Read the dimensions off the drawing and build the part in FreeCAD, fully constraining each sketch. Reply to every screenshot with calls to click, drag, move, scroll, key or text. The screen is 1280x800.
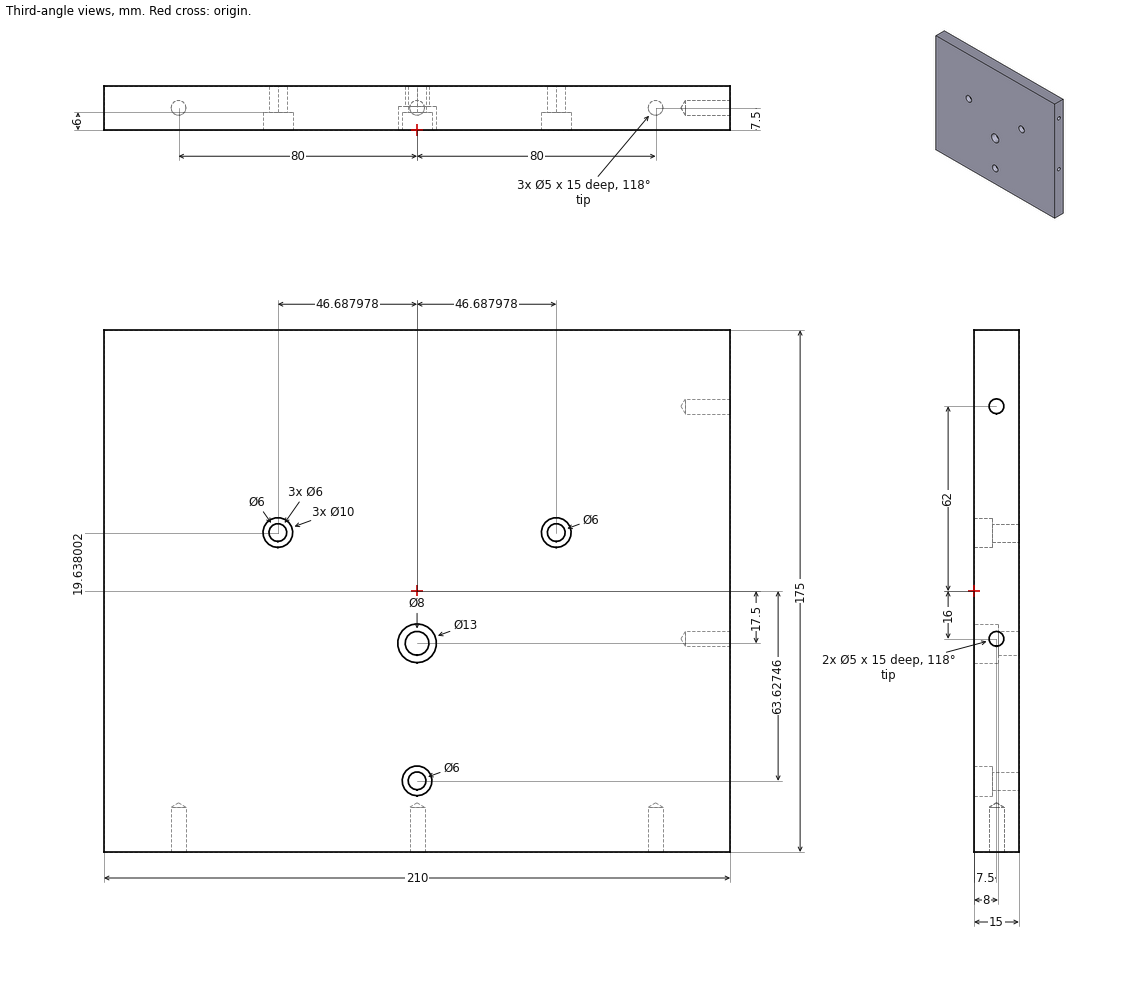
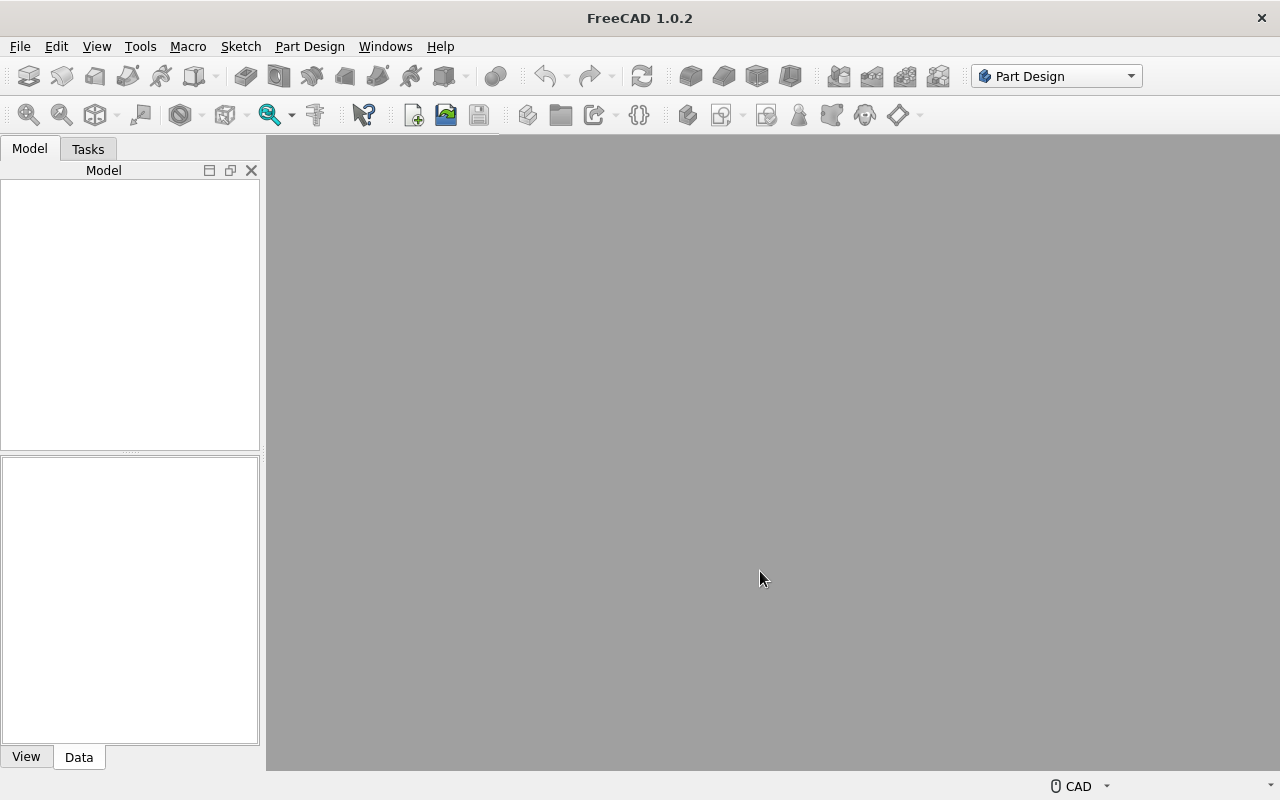
click(413, 116)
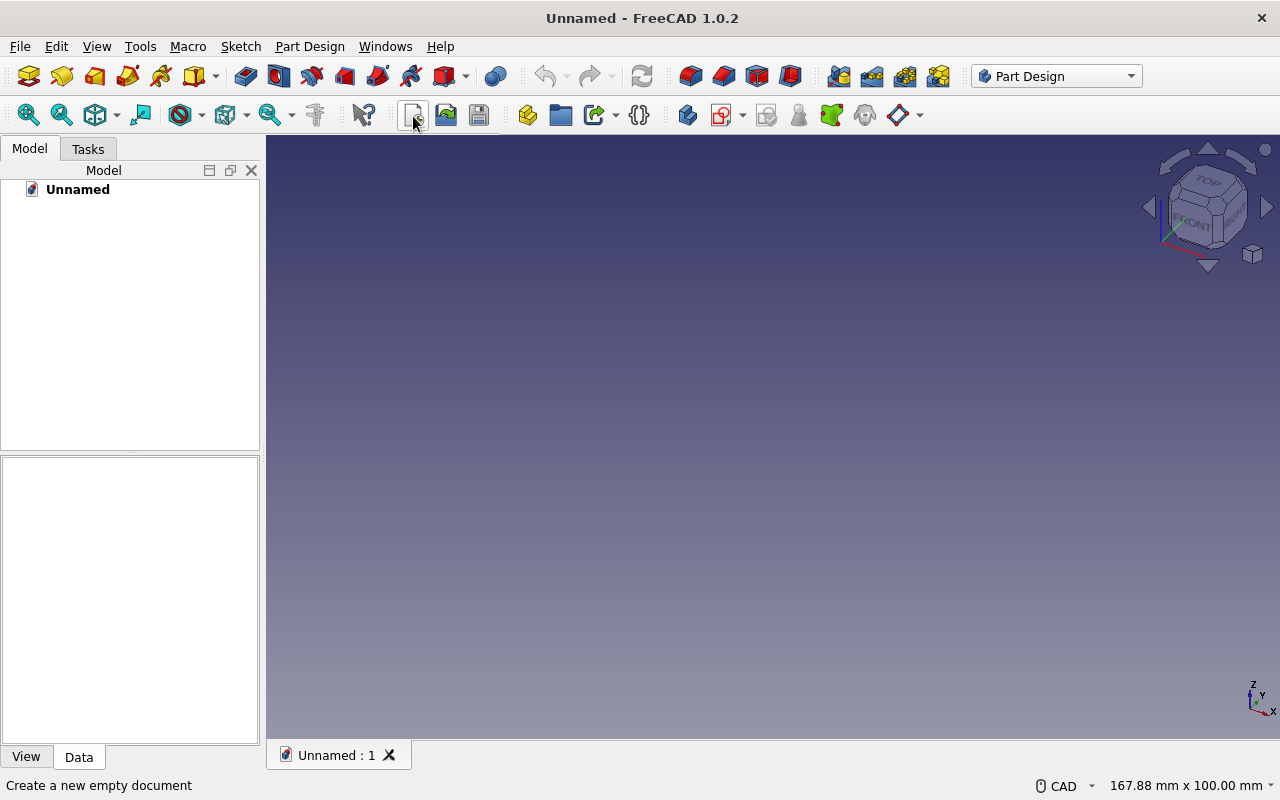
click(720, 116)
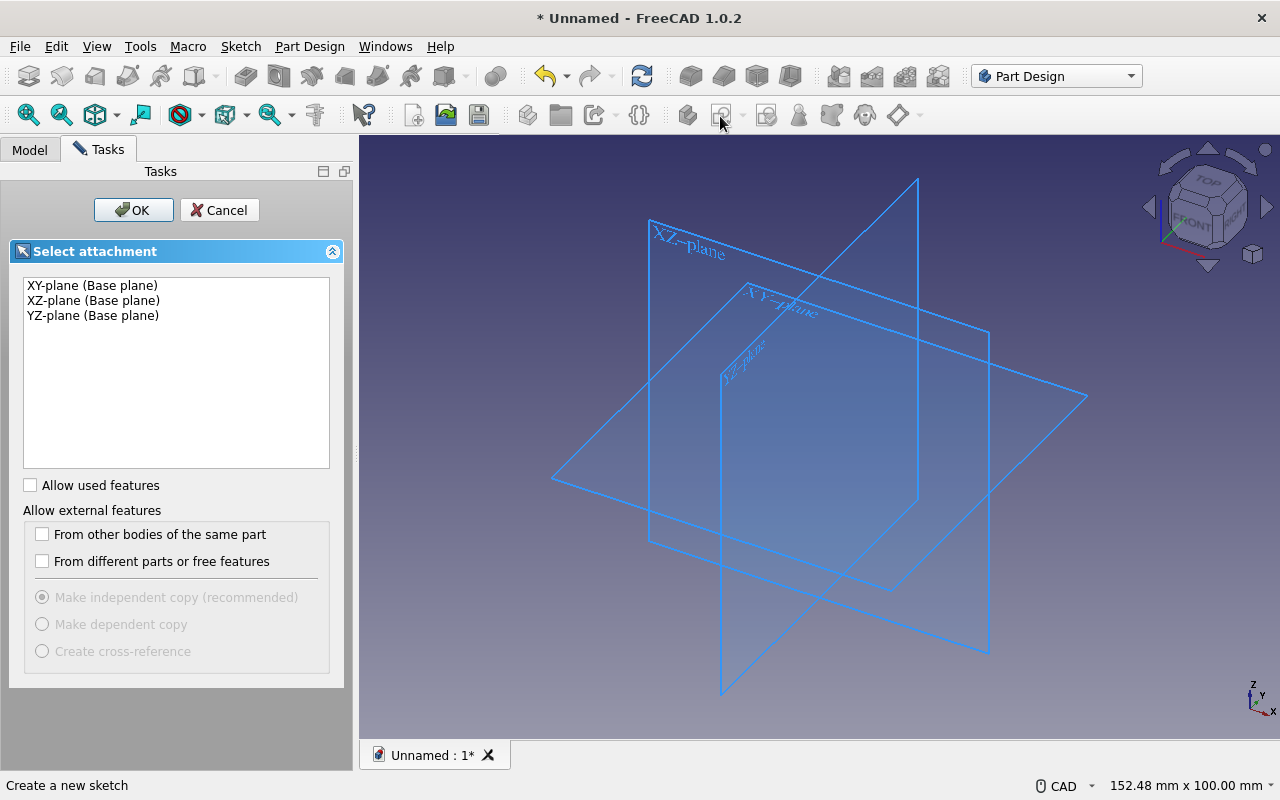
click(84, 300)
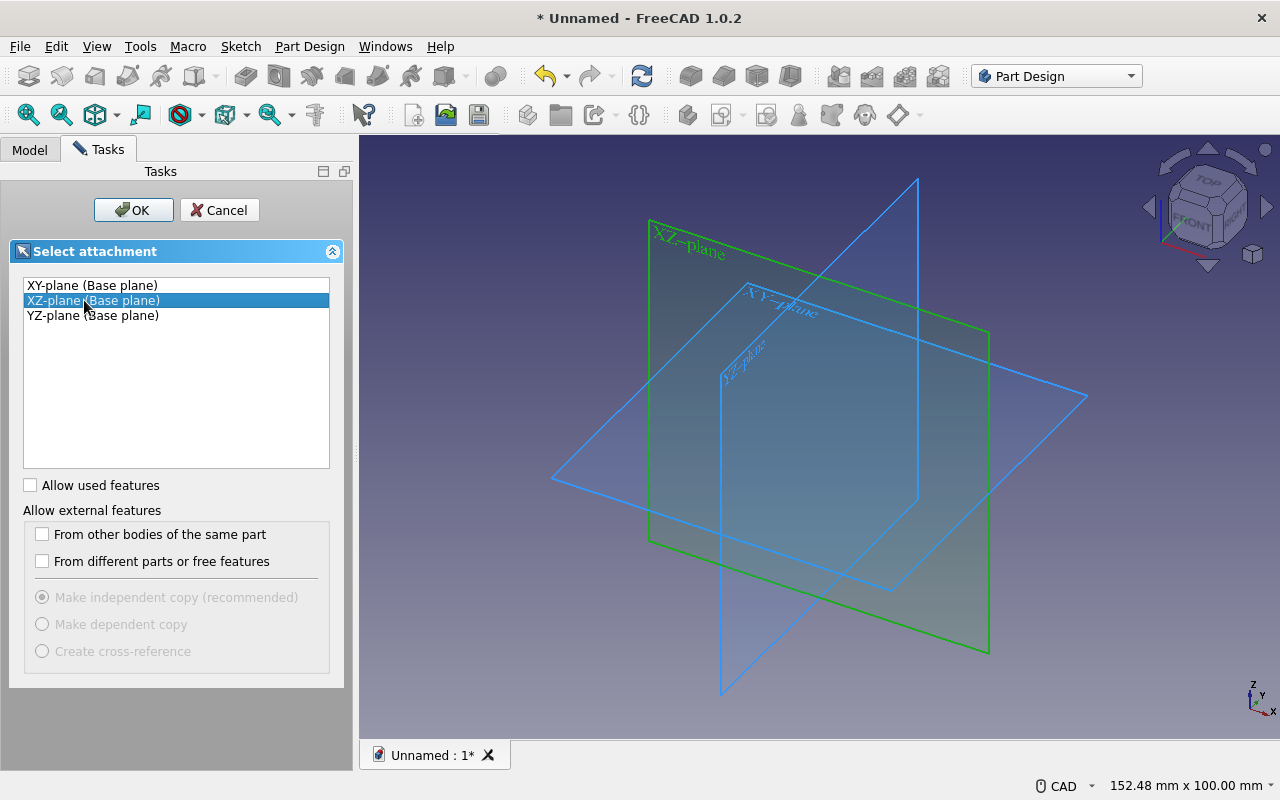
click(134, 210)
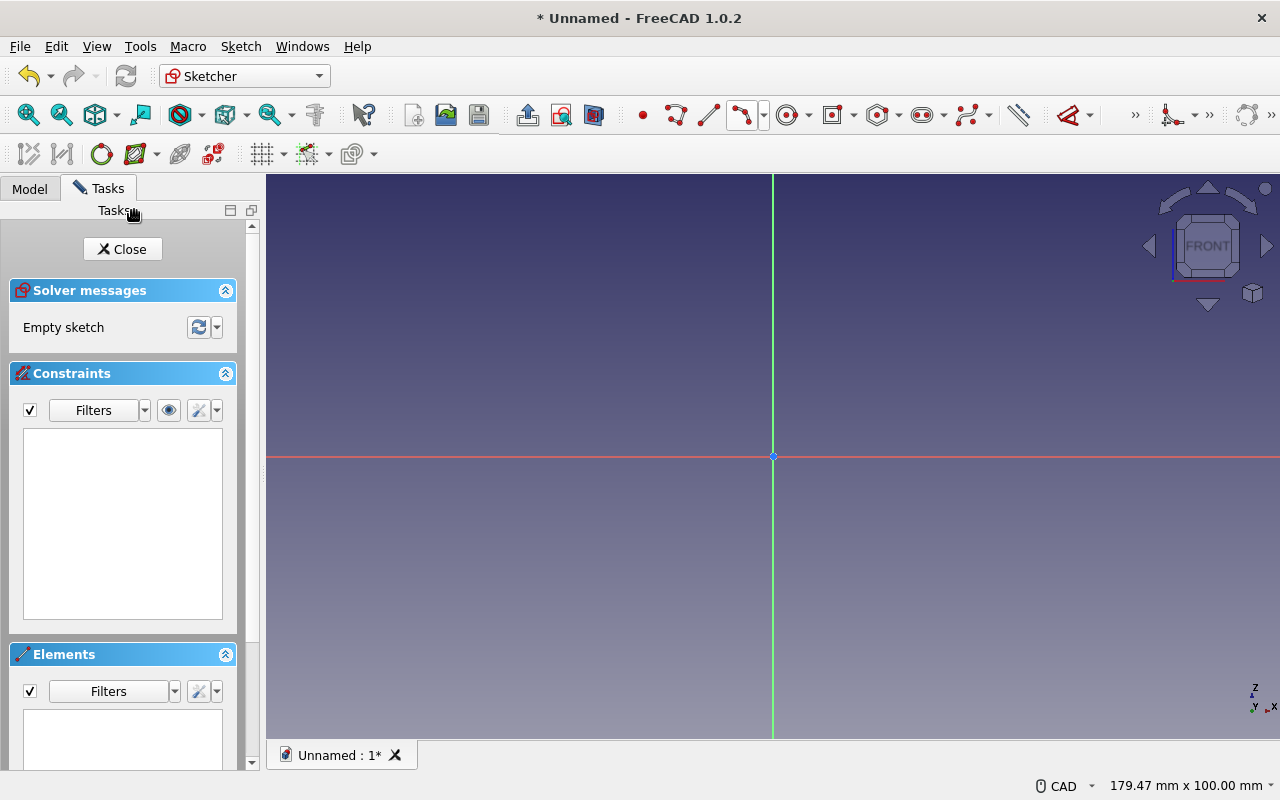
scroll(665, 456, down, 5)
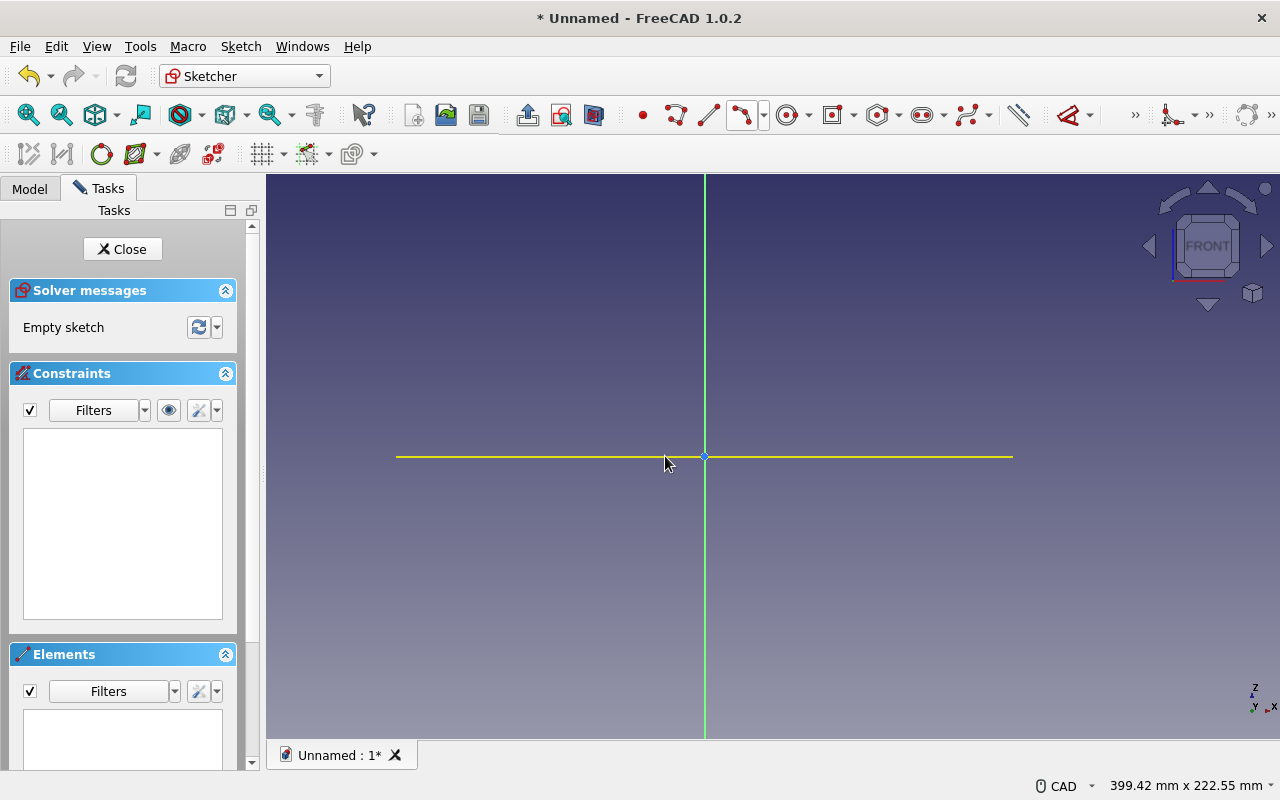
click(832, 116)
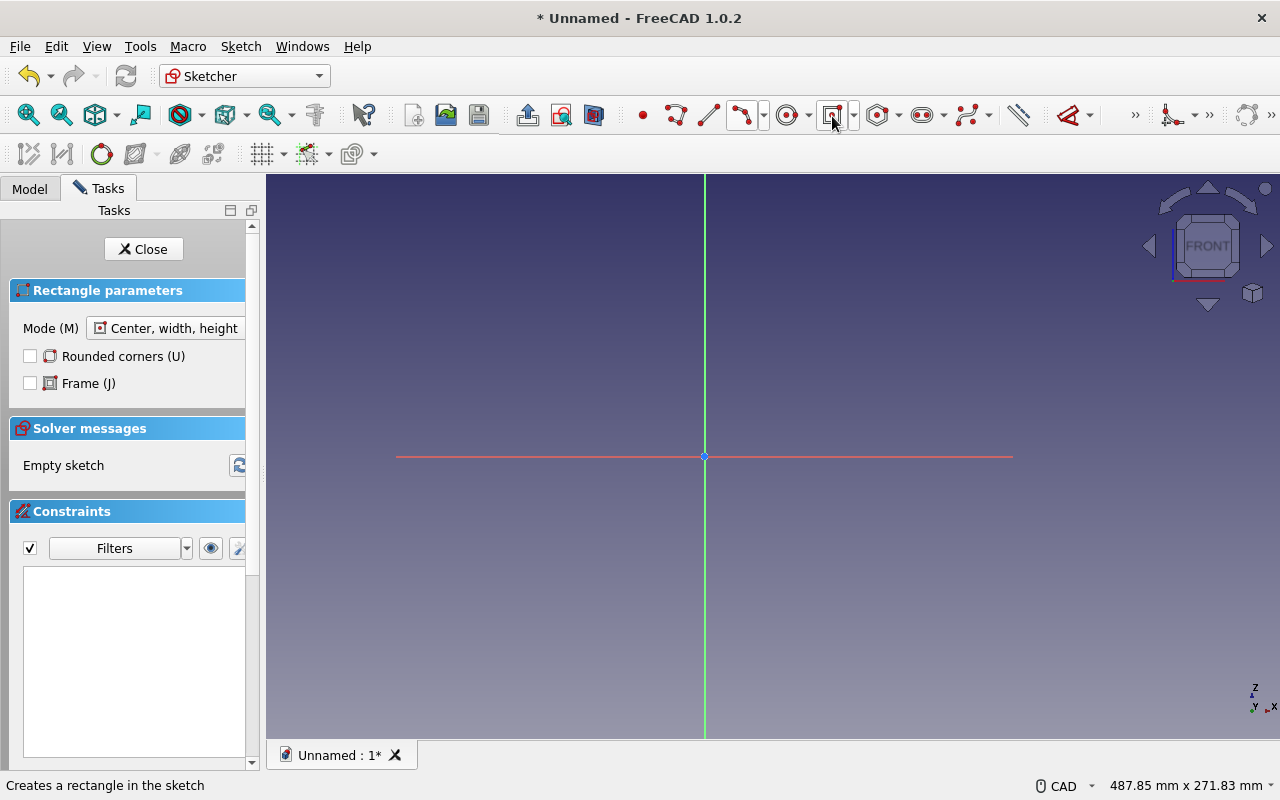
click(705, 456)
click(923, 275)
key(Escape)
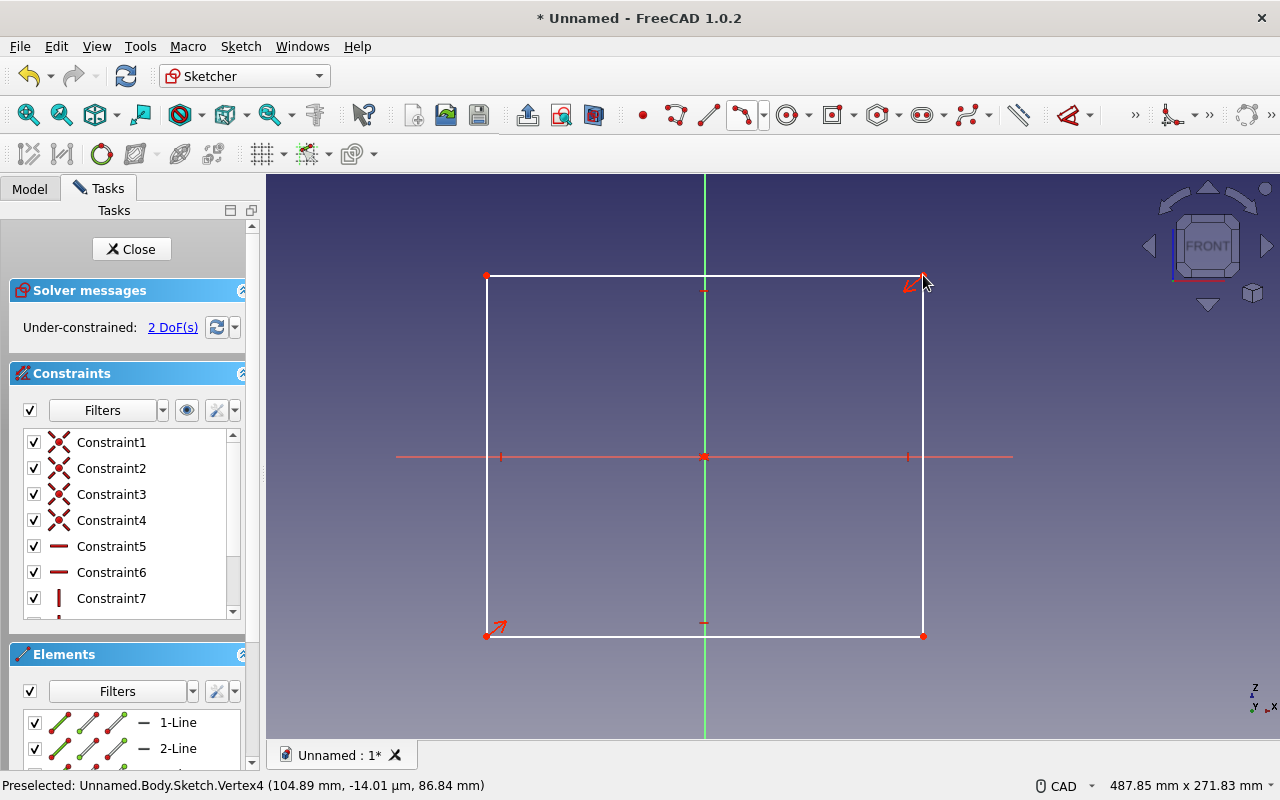
click(618, 637)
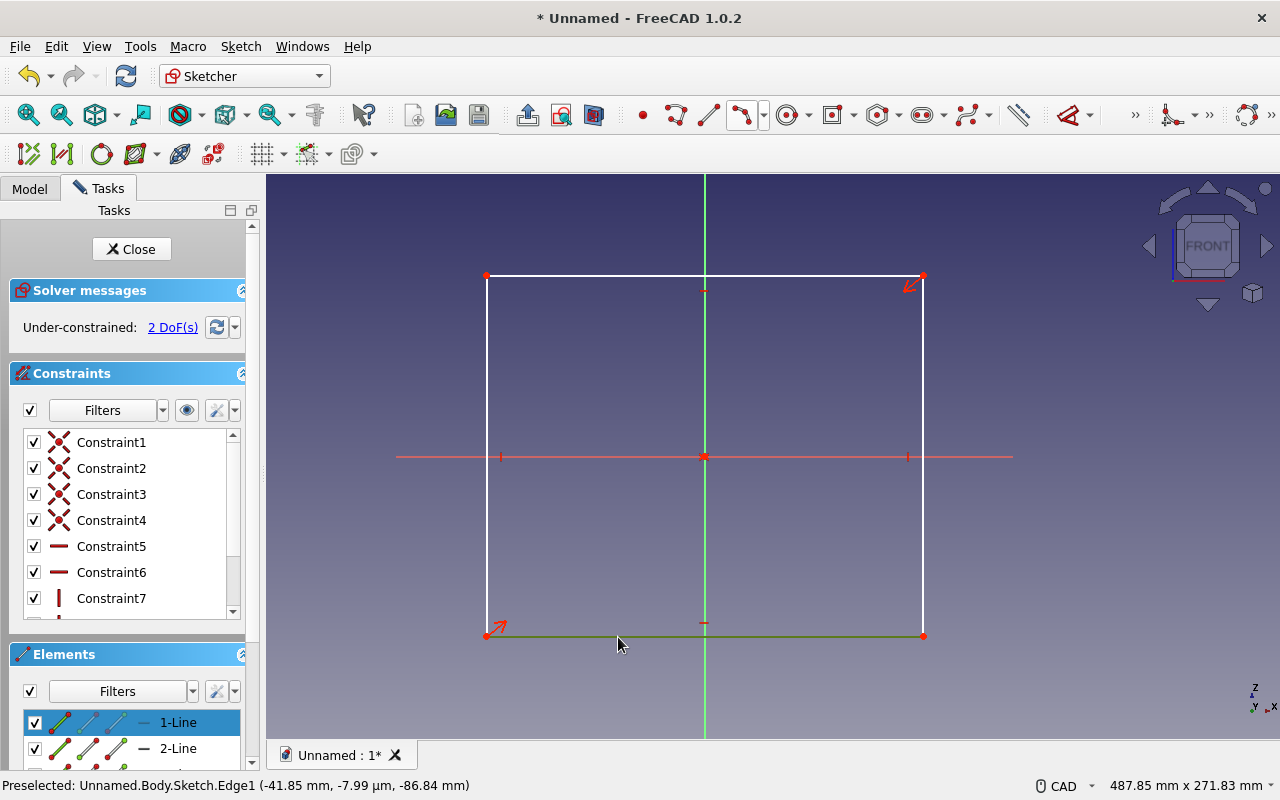
key(l)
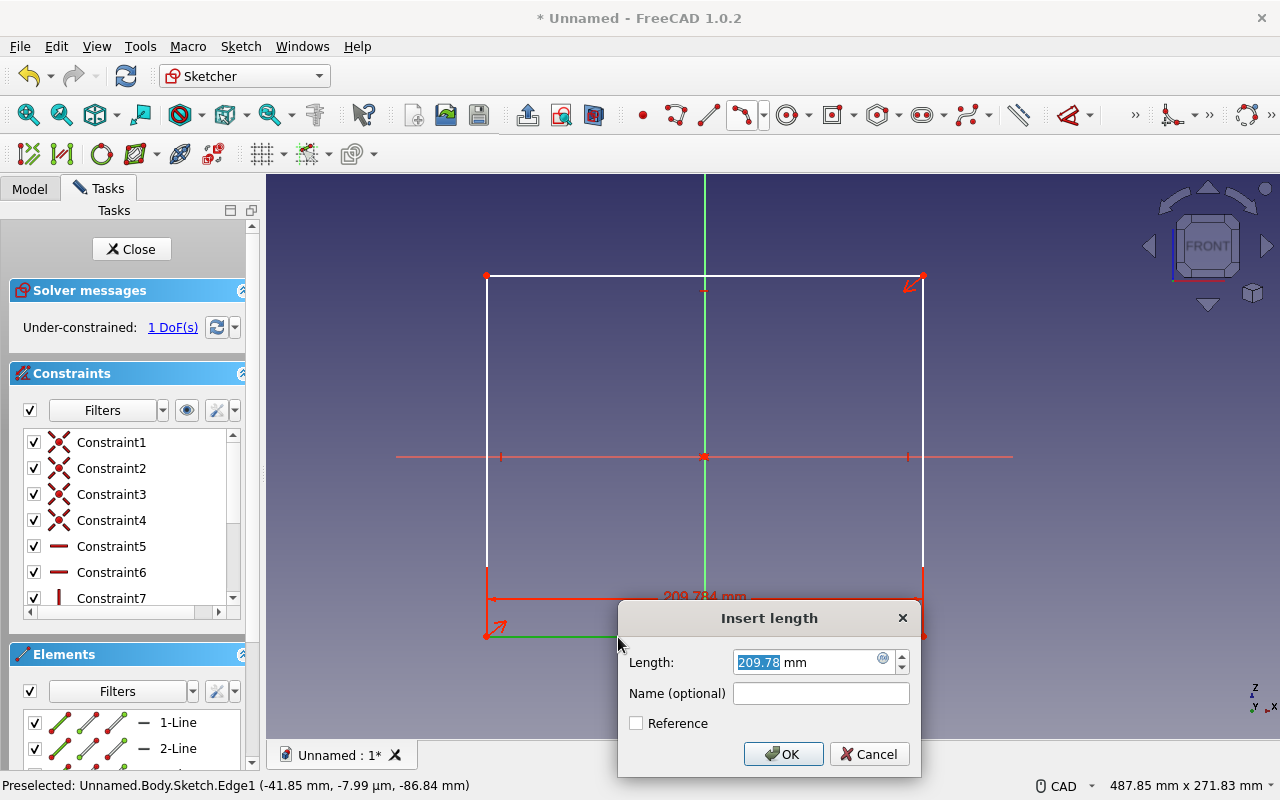
text(210)
key(Return)